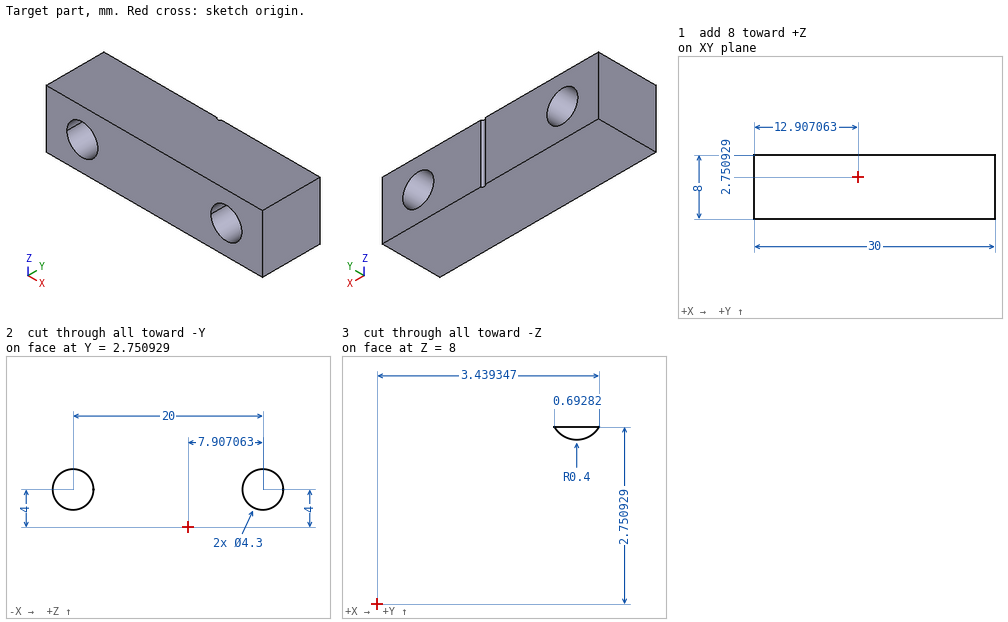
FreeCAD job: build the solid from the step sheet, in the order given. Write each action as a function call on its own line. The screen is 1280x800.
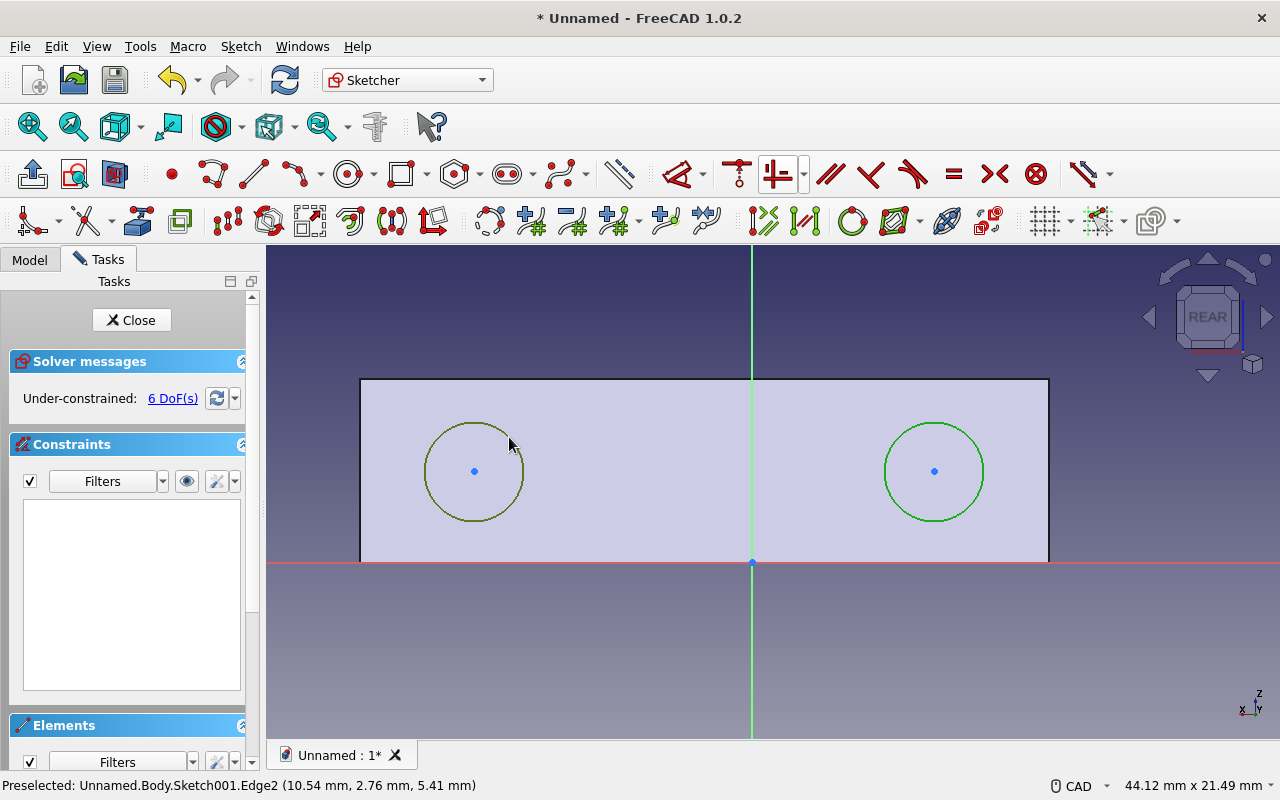
key(e)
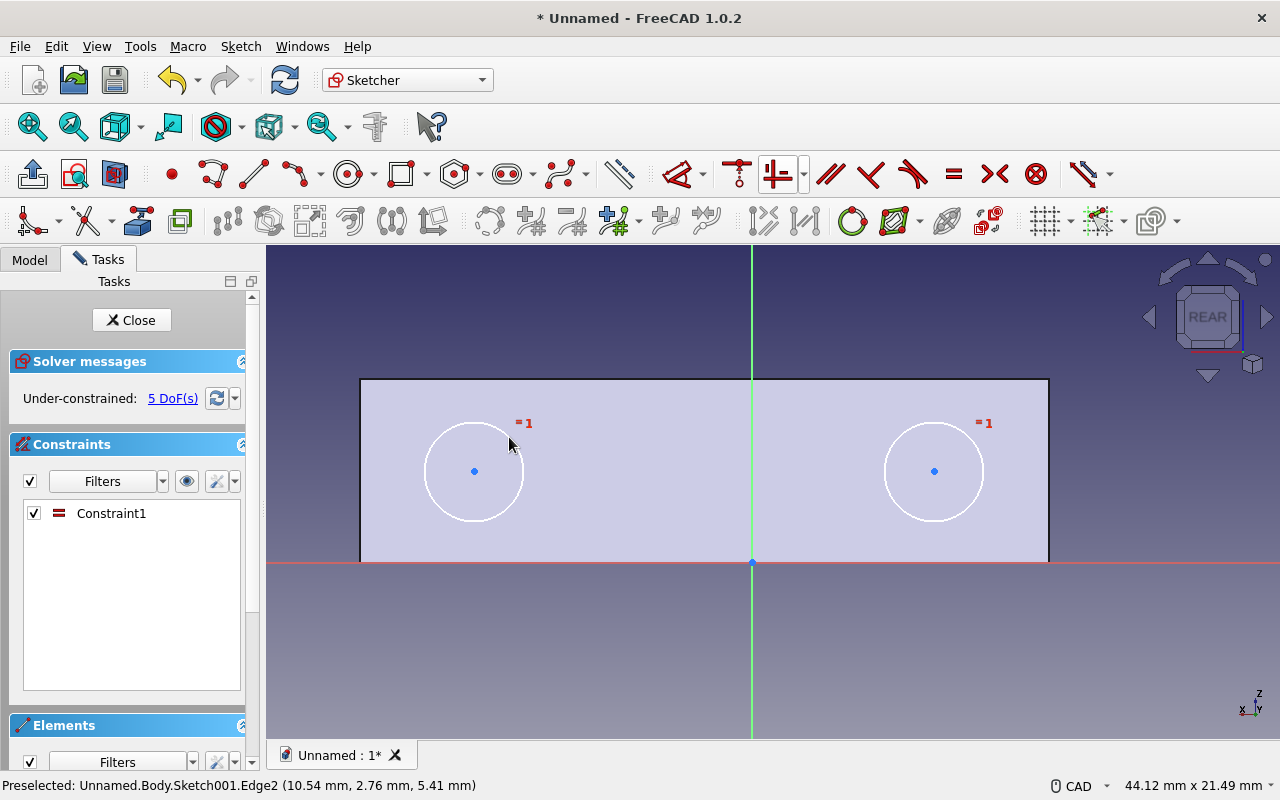
key(d)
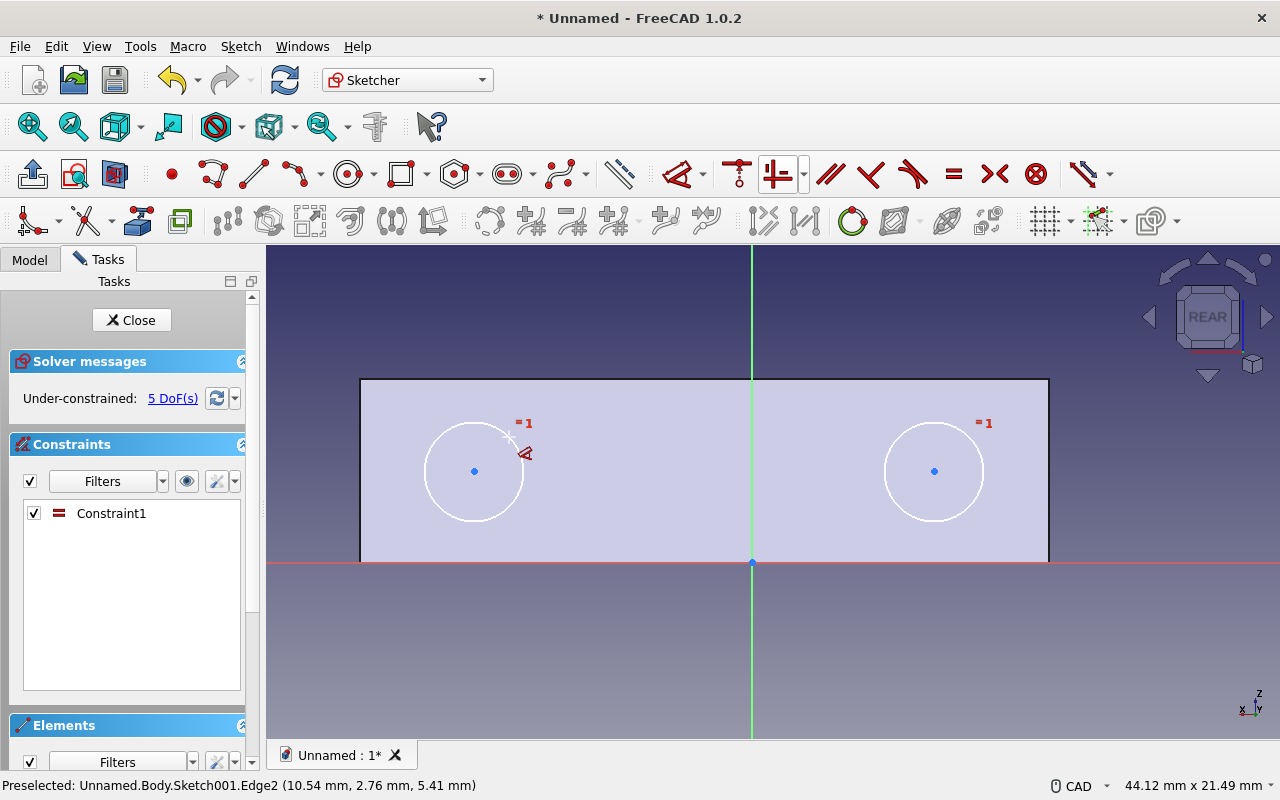
click(969, 437)
click(992, 414)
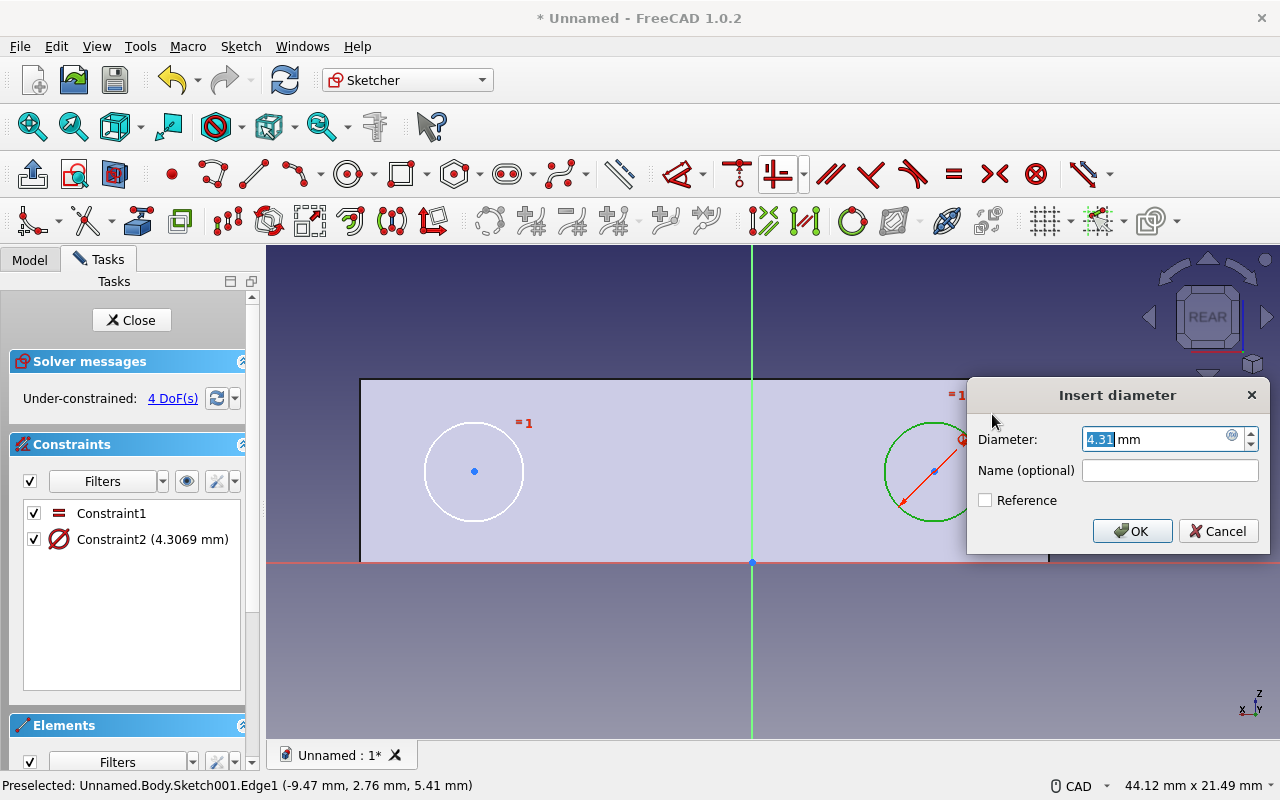
text(4.3)
key(Return)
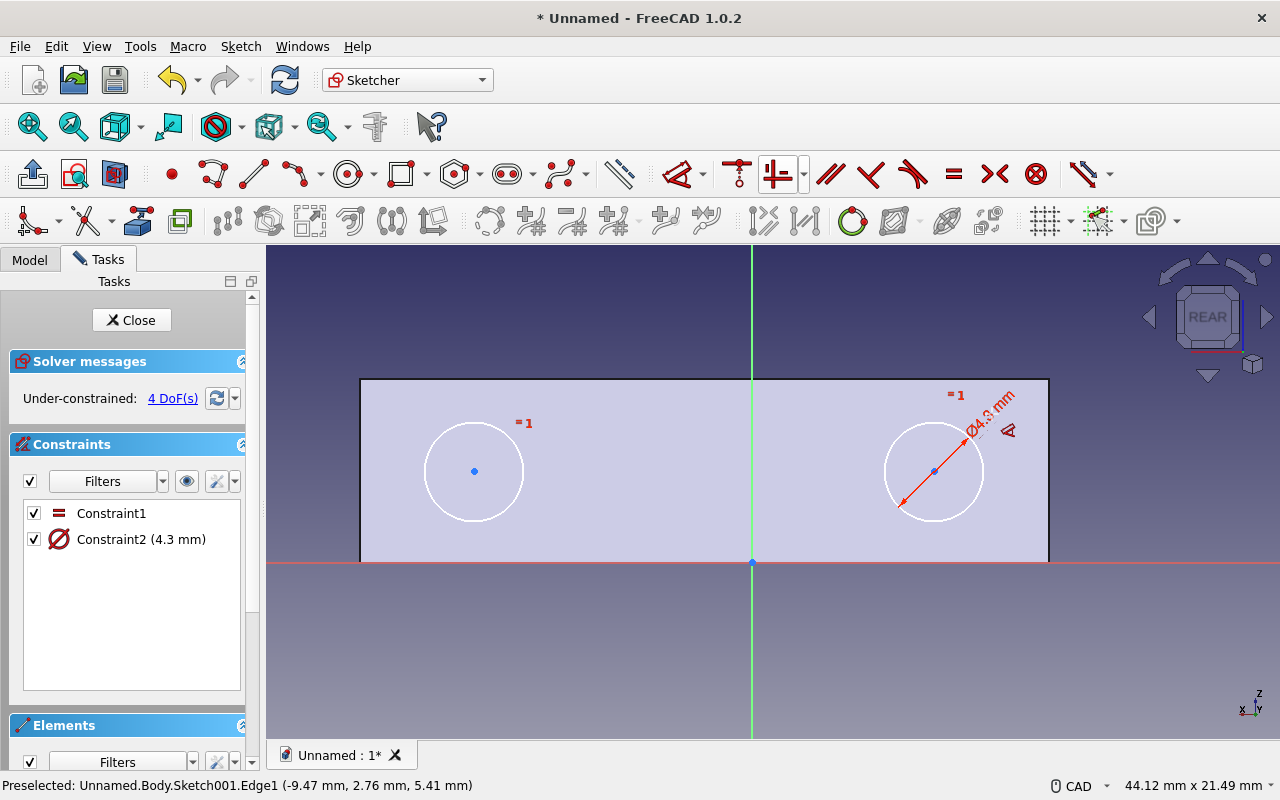
click(934, 472)
click(968, 538)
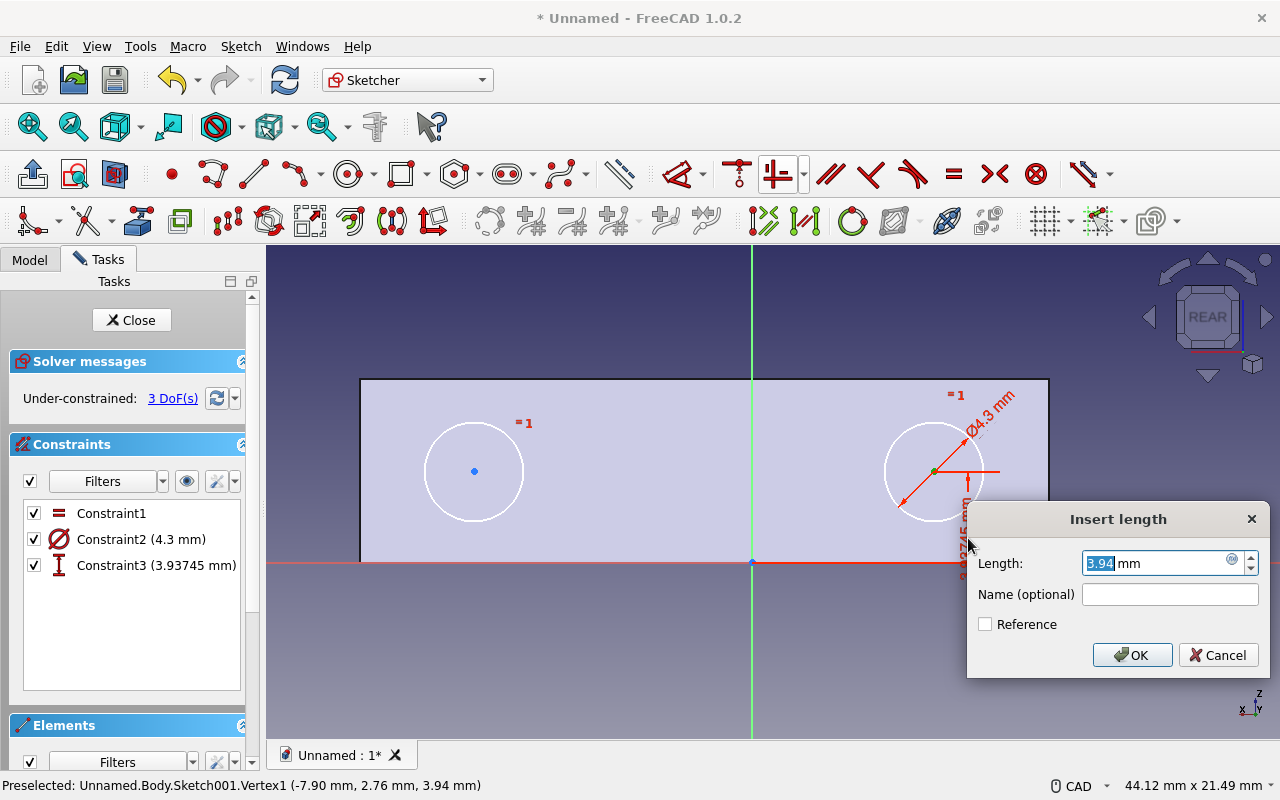
text(4)
key(Return)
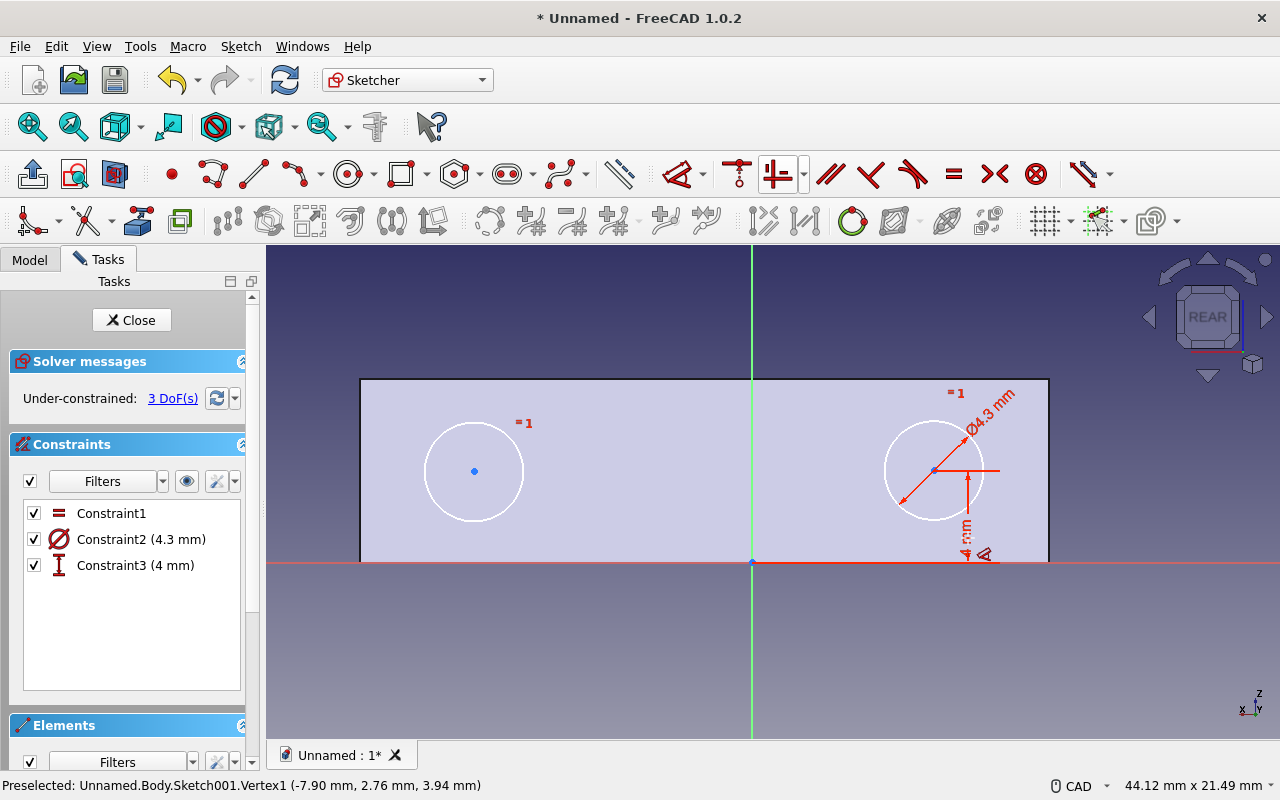
click(474, 472)
click(440, 538)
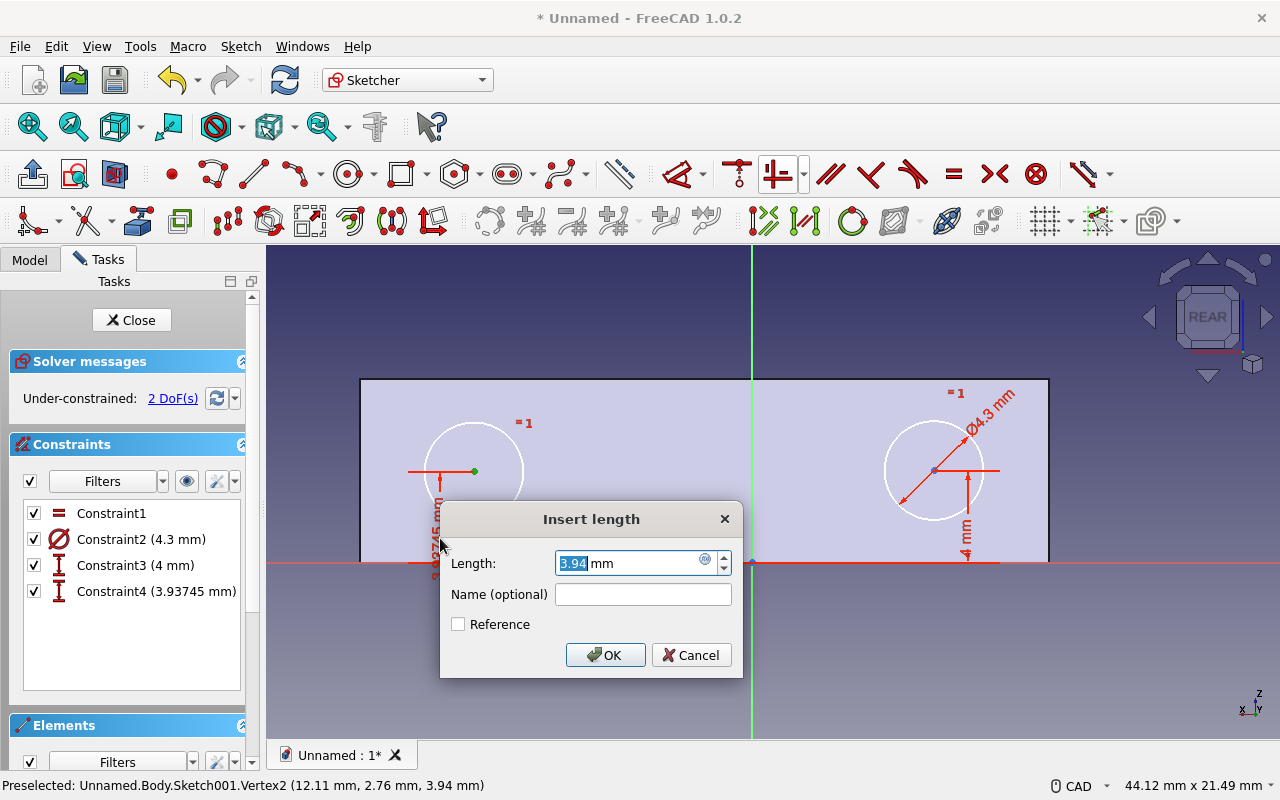
text(4)
key(Return)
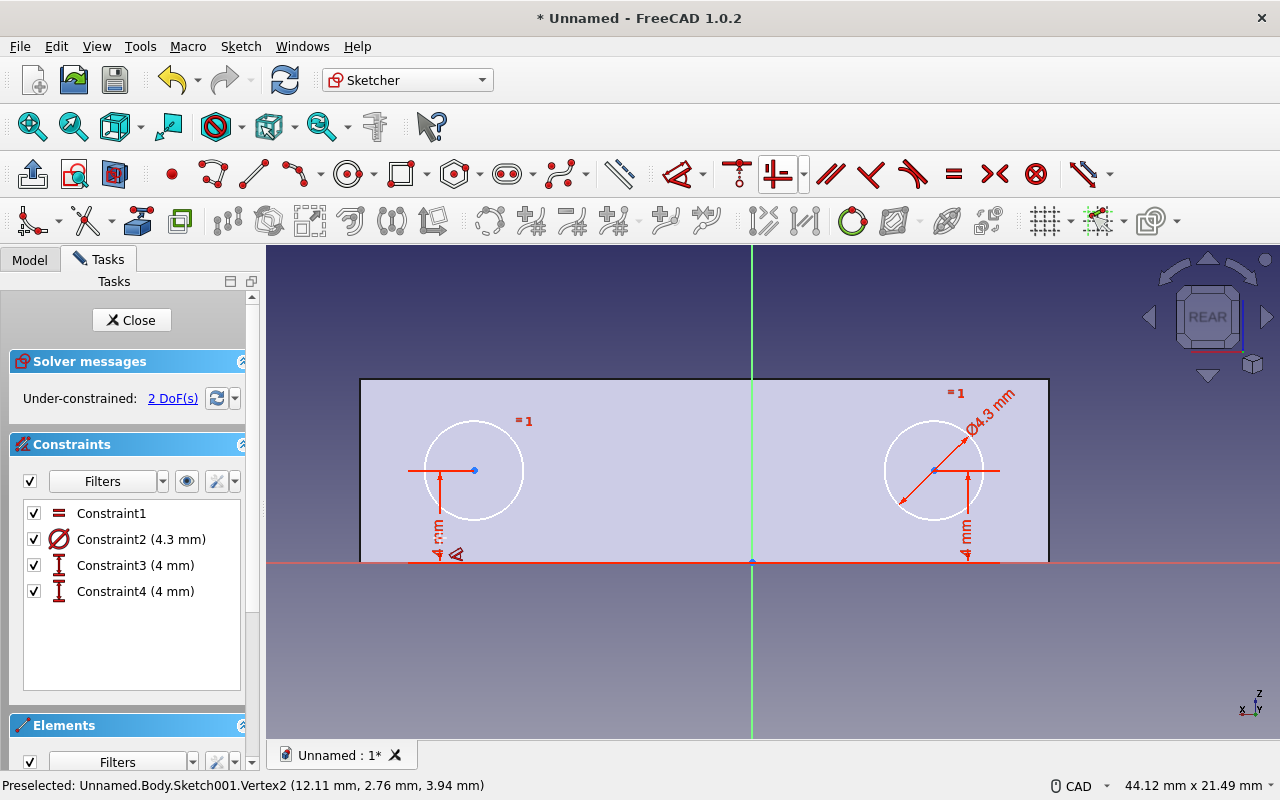
click(934, 471)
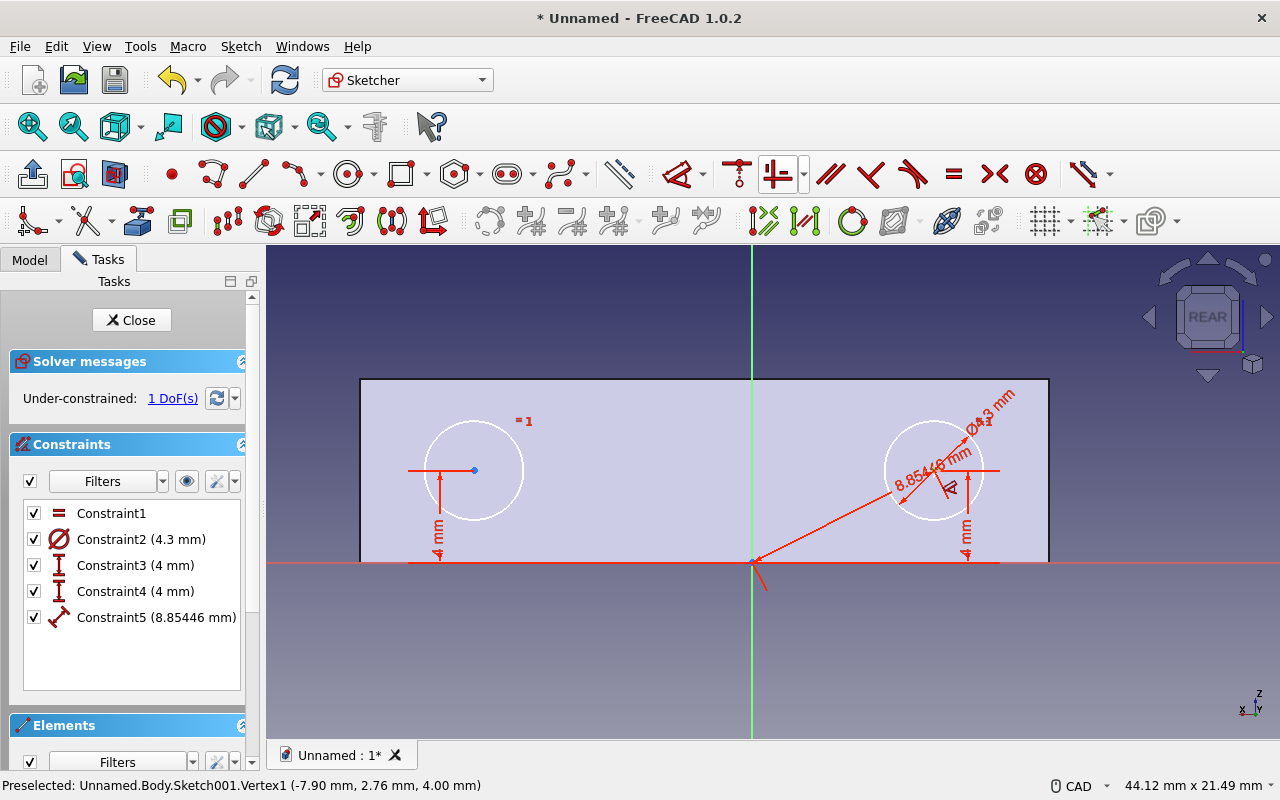
click(474, 471)
click(704, 437)